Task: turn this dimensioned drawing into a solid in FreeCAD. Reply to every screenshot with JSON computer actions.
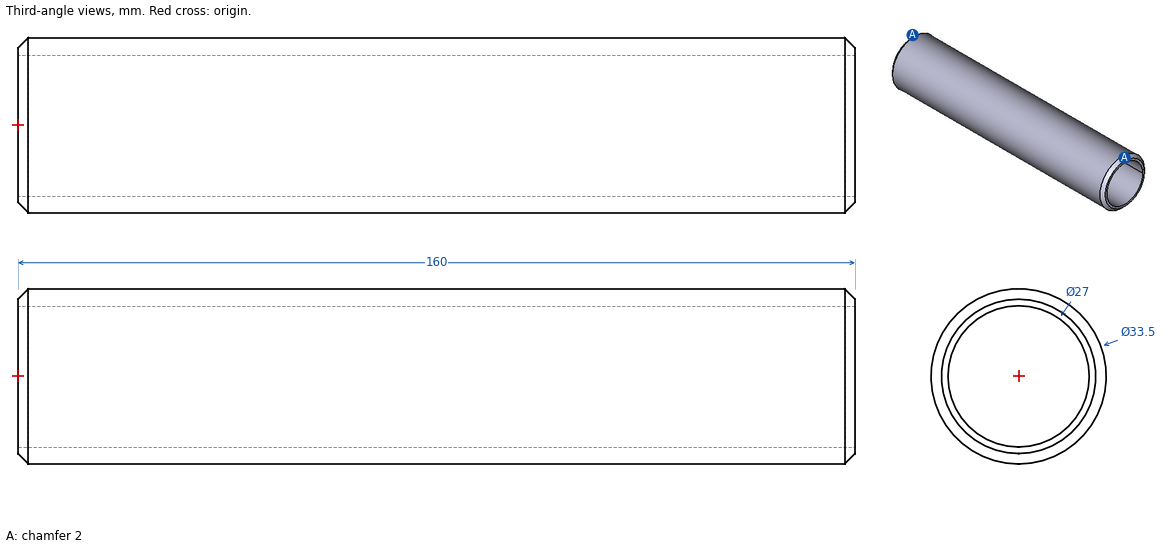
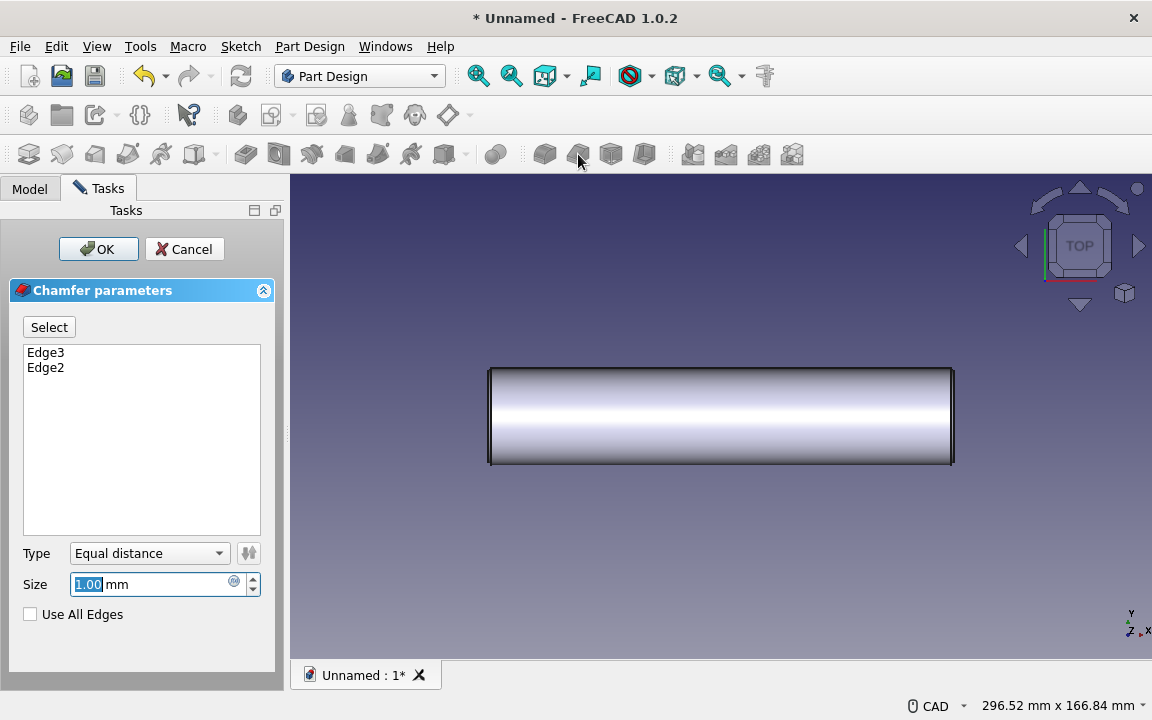
{"action": "type", "text": "2"}
{"action": "key", "text": "Tab"}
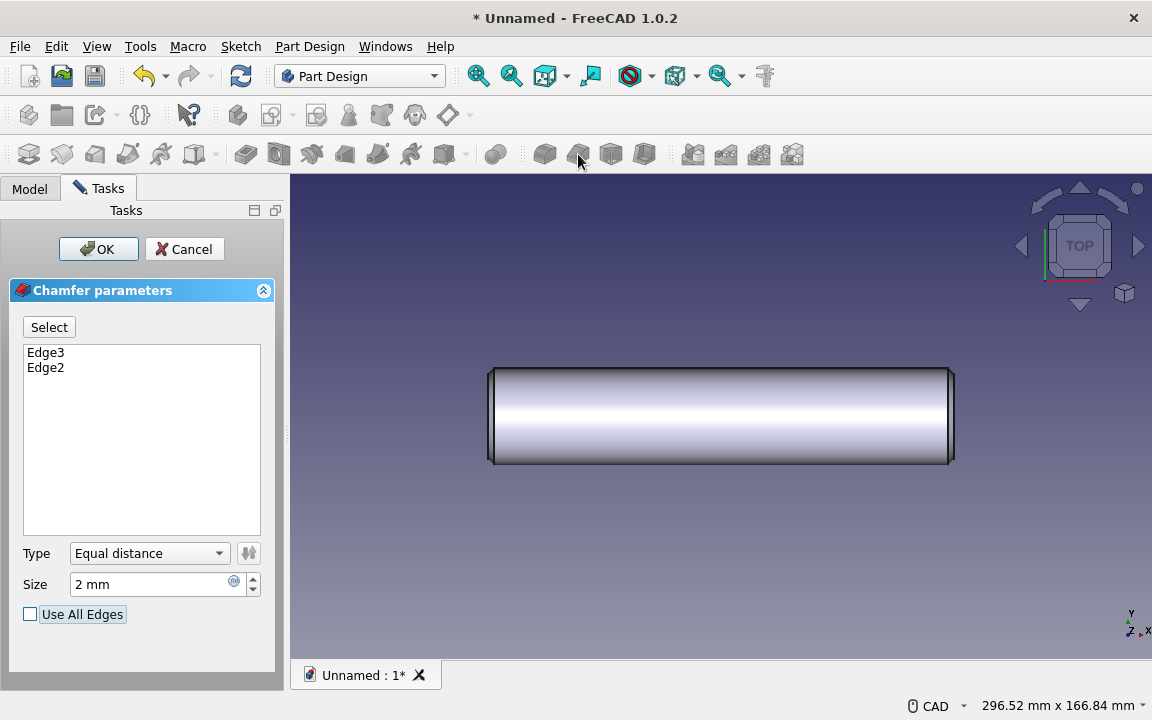
{"action": "left_click", "coordinate": [99, 249]}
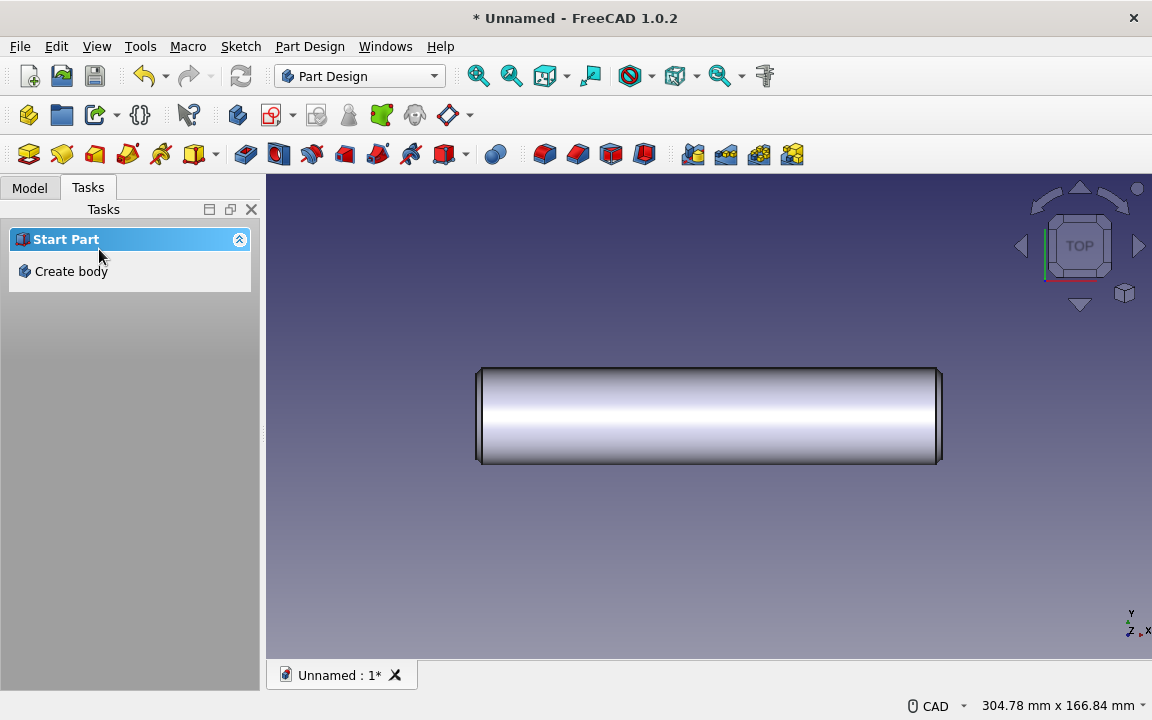
{"action": "key", "text": "0"}